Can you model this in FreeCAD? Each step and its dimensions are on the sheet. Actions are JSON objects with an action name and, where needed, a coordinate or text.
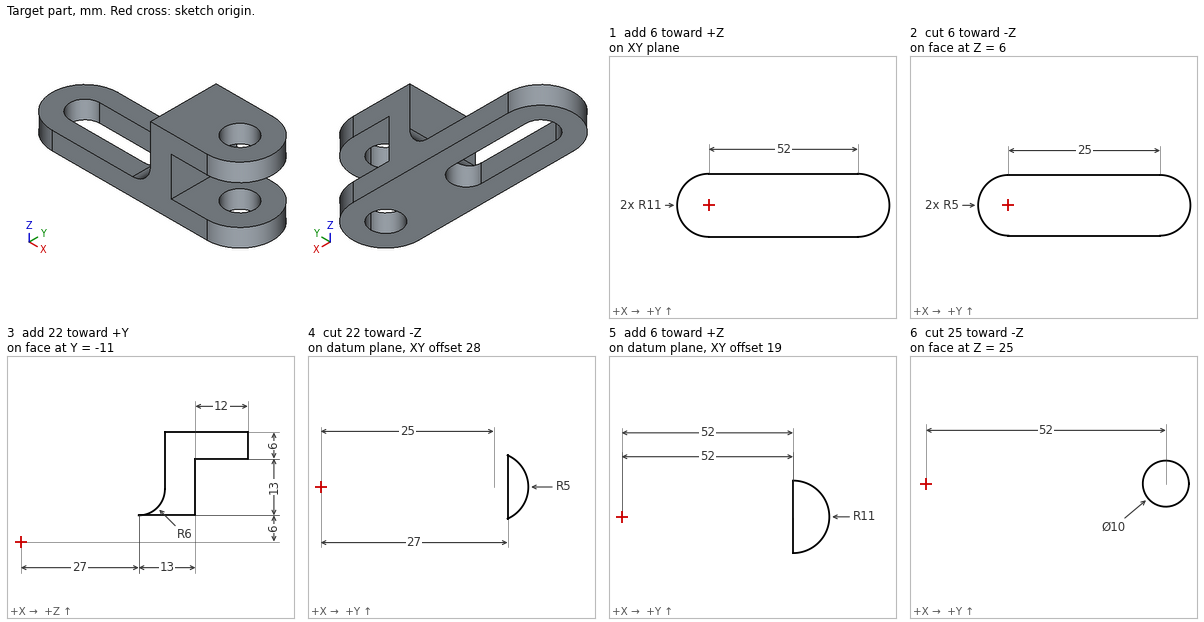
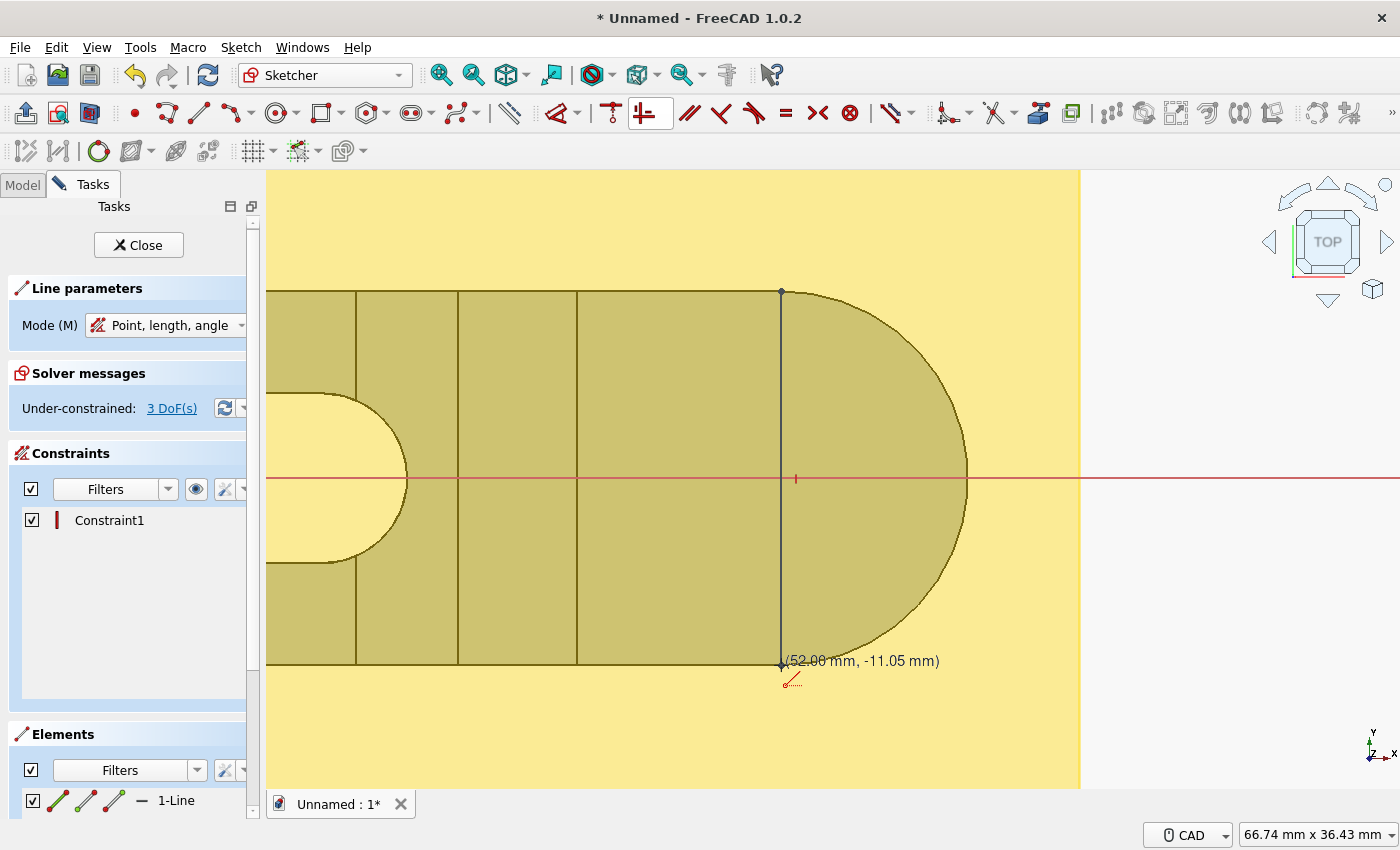
{"action": "left_click", "coordinate": [232, 114]}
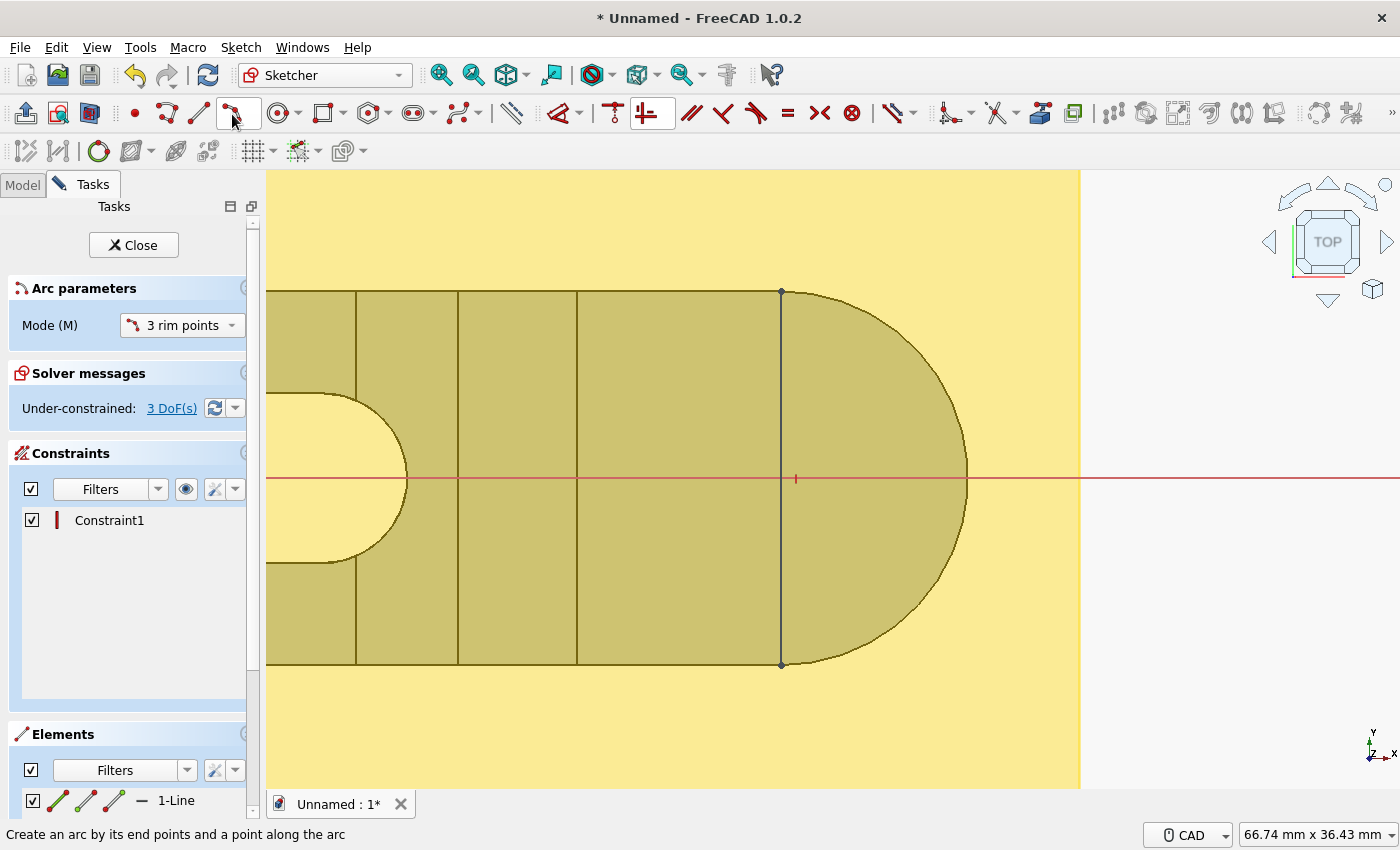
{"action": "left_click", "coordinate": [781, 666]}
{"action": "left_click", "coordinate": [781, 292]}
{"action": "left_click", "coordinate": [959, 536]}
{"action": "key", "text": "Escape"}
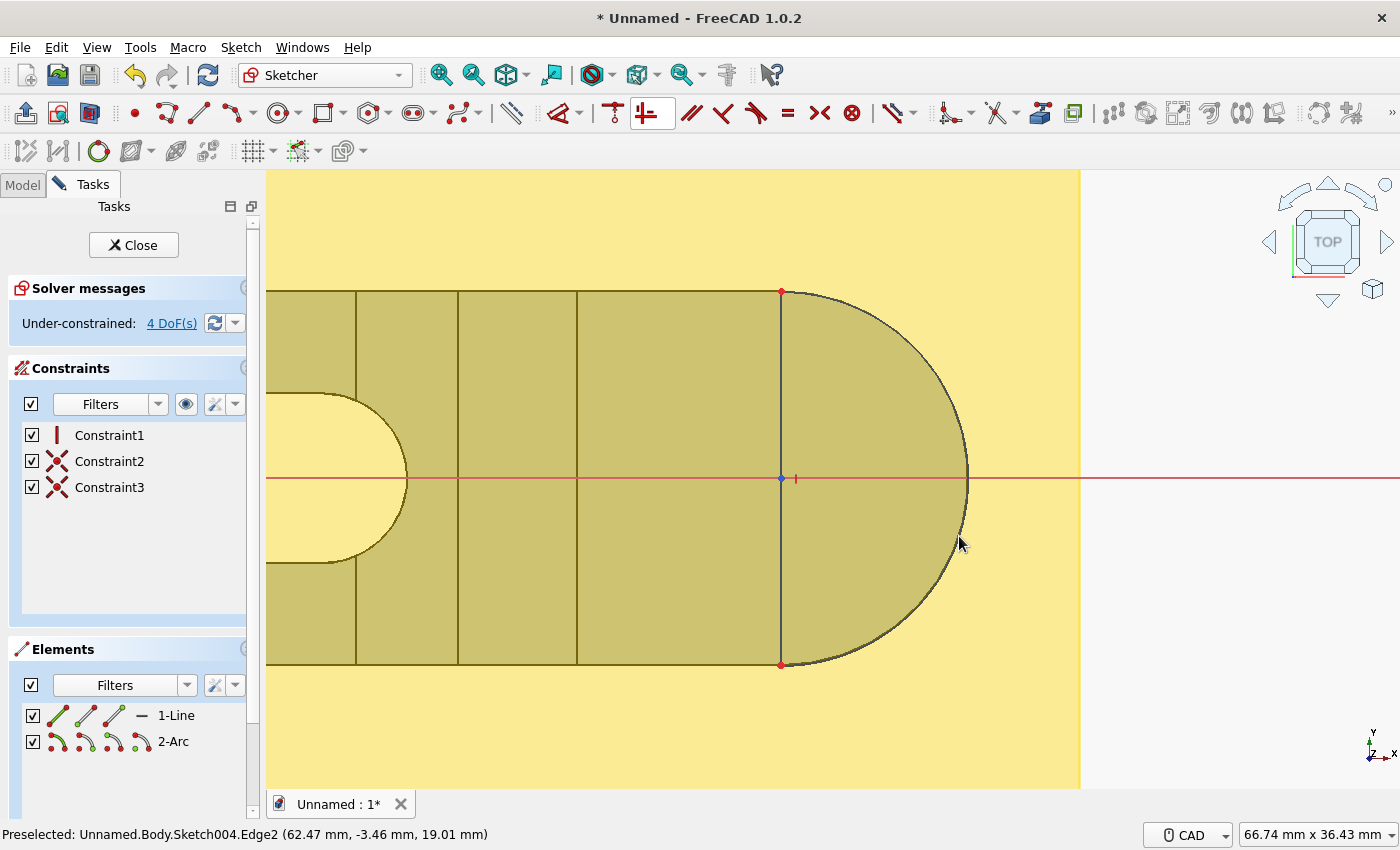
{"action": "left_click", "coordinate": [781, 479]}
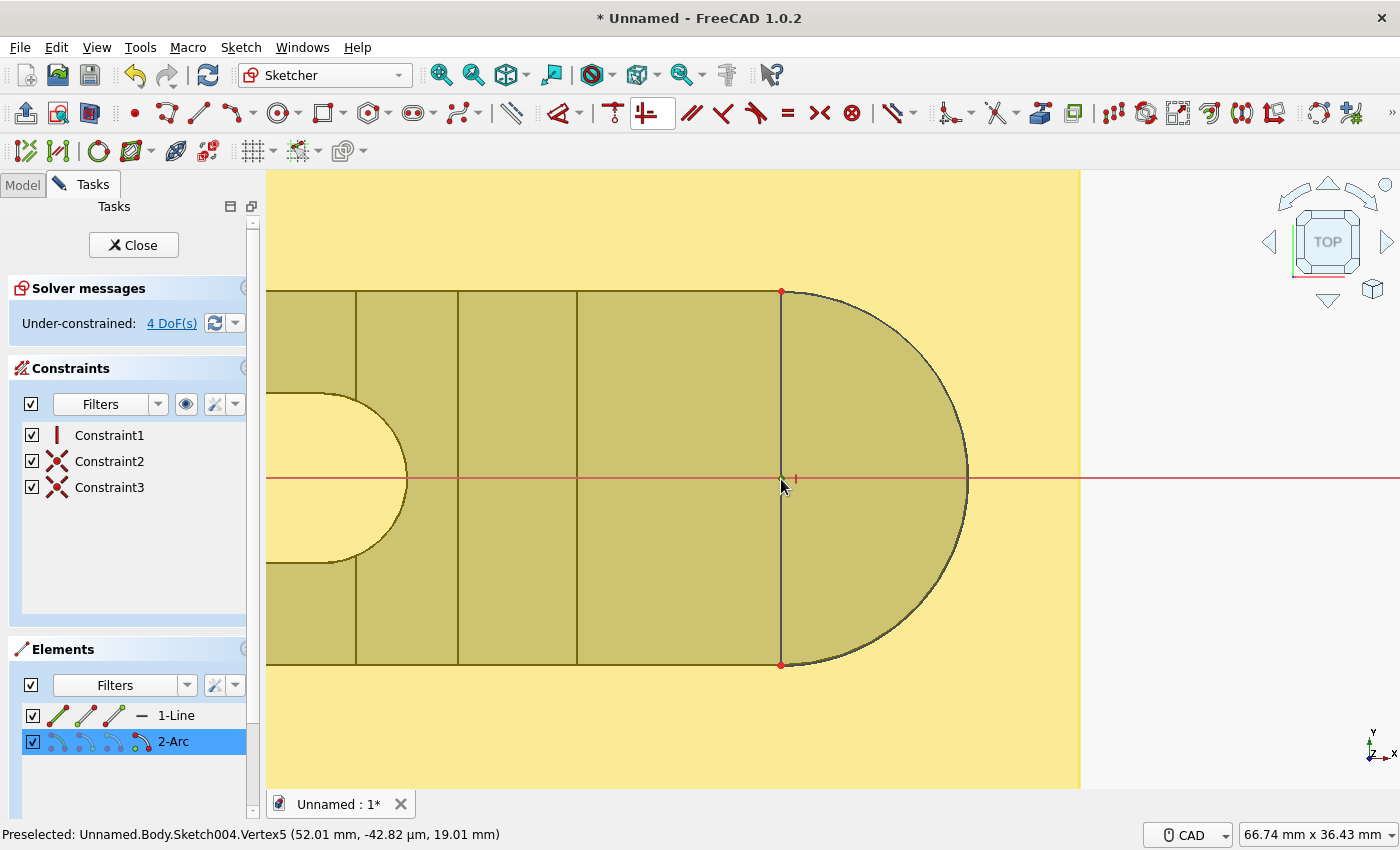
{"action": "left_click", "coordinate": [361, 478]}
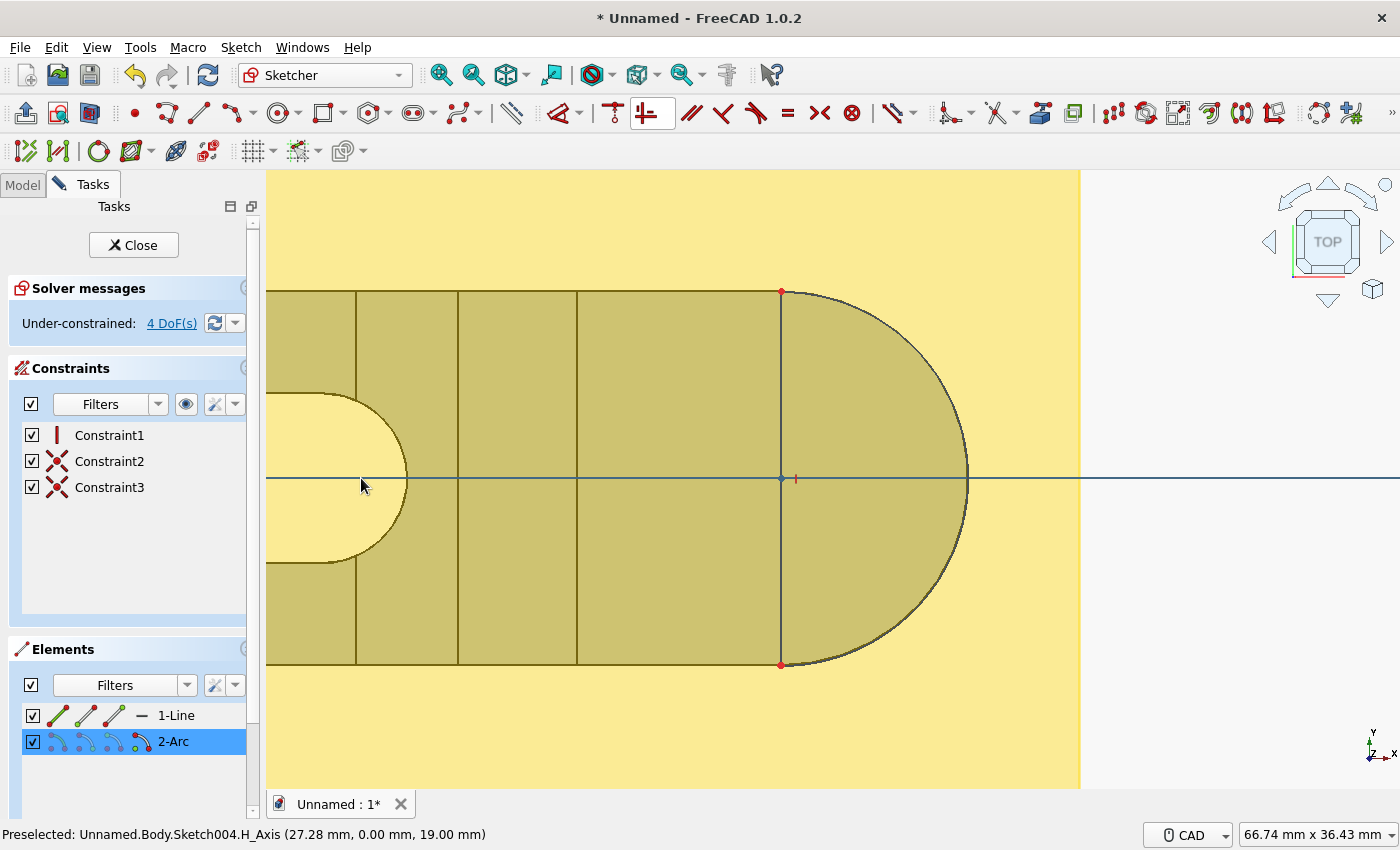
{"action": "key", "text": "c"}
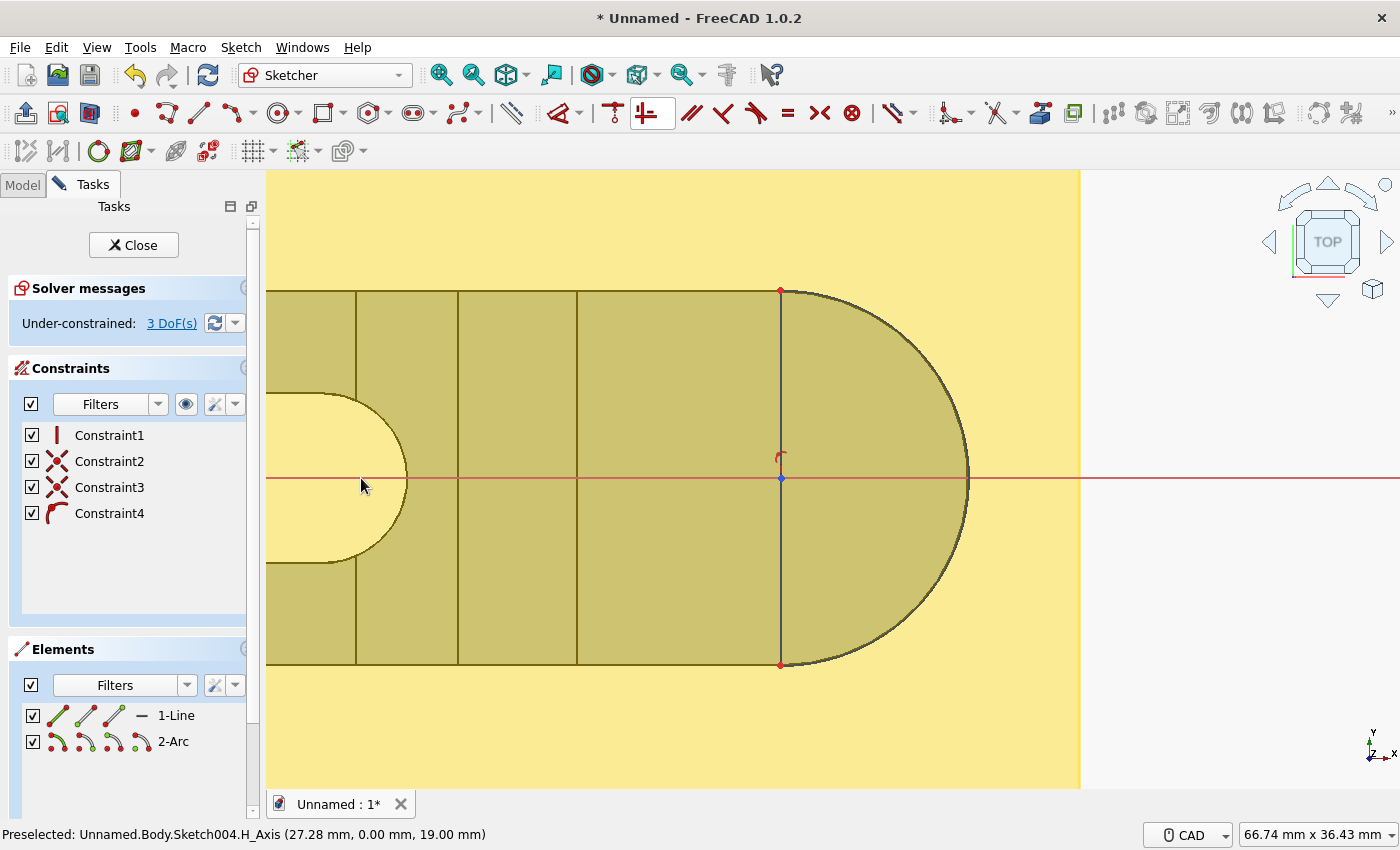
{"action": "left_click", "coordinate": [558, 114]}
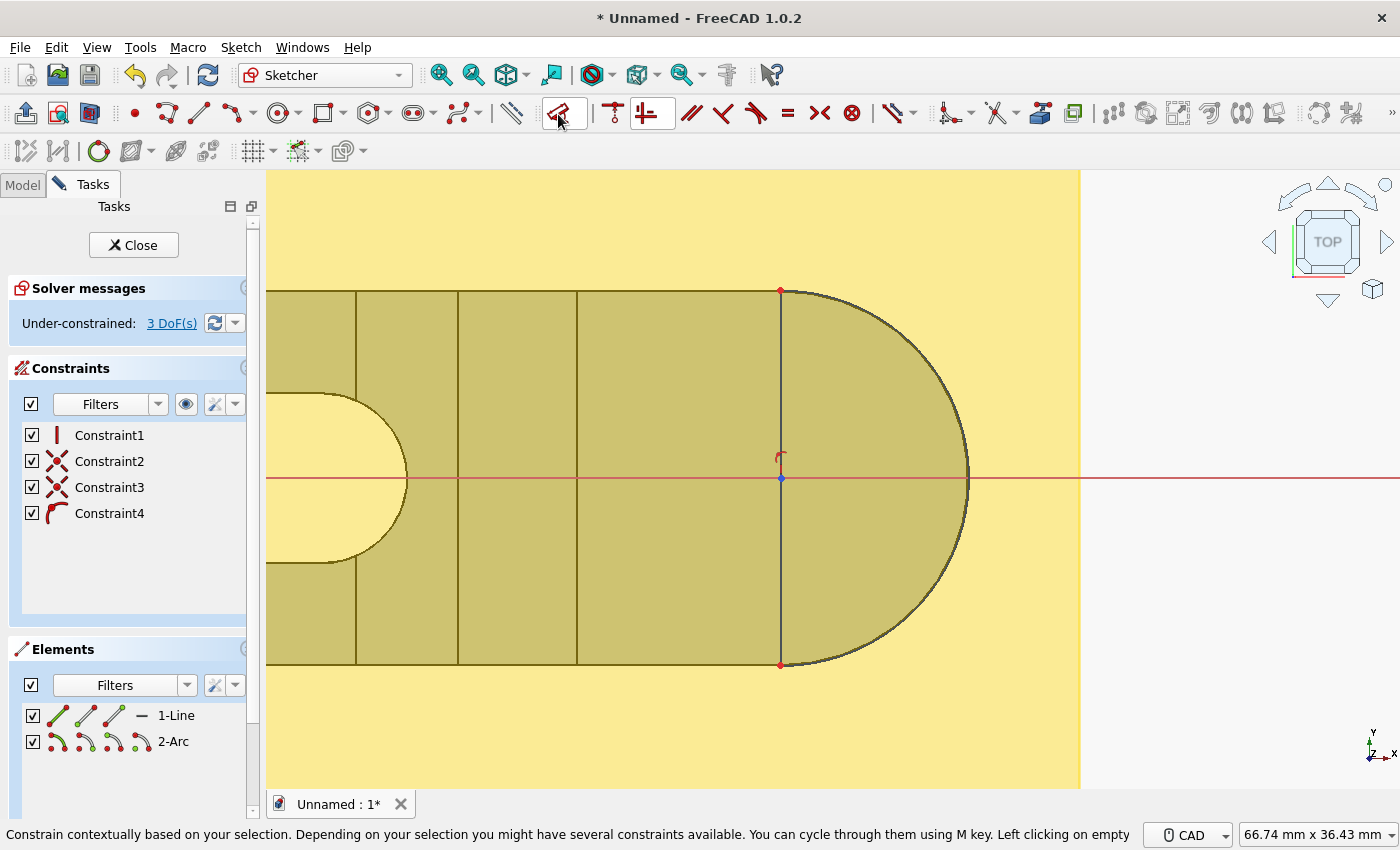
{"action": "left_click", "coordinate": [933, 589]}
{"action": "left_click", "coordinate": [959, 608]}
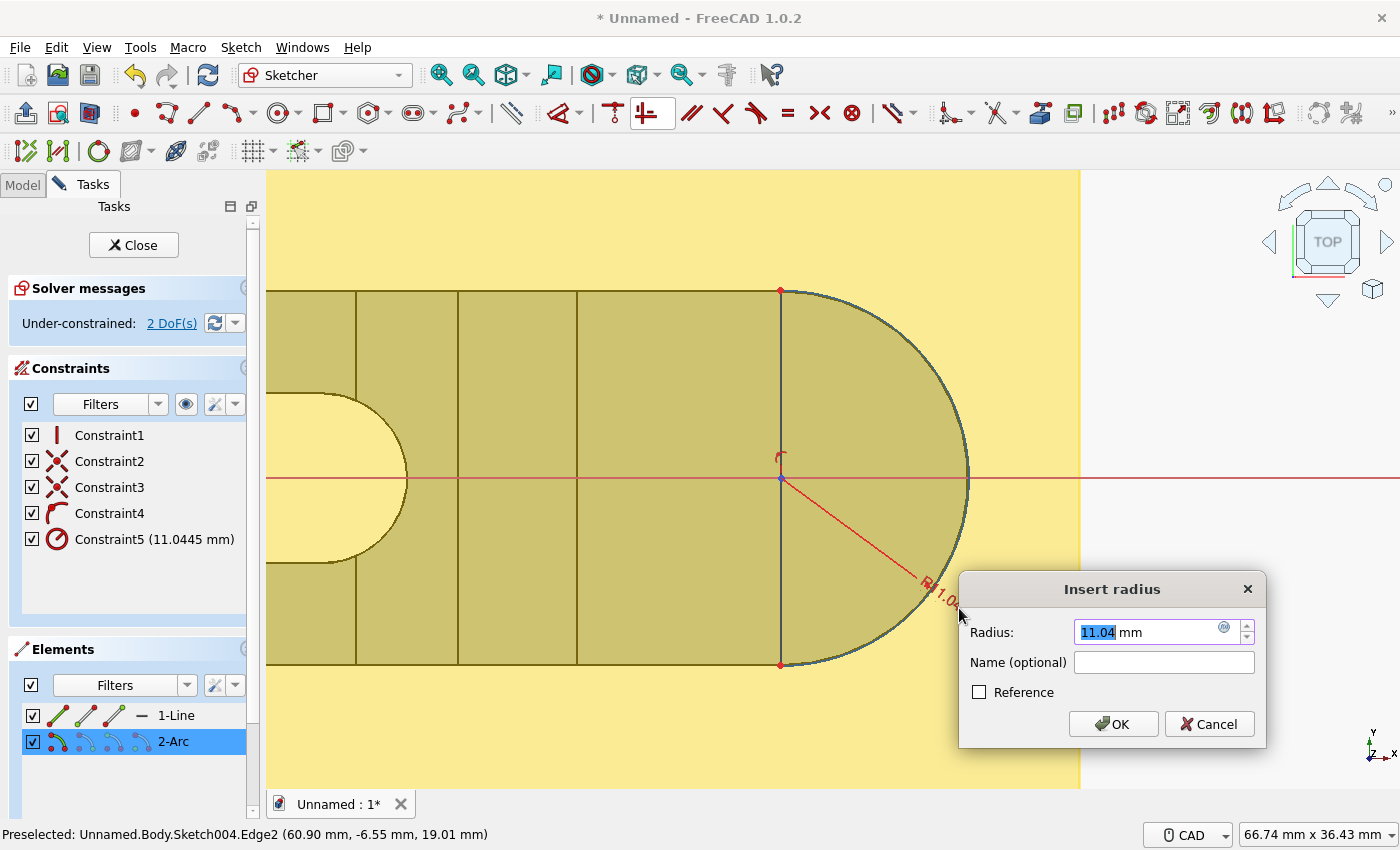
{"action": "type", "text": "11"}
{"action": "key", "text": "Return"}